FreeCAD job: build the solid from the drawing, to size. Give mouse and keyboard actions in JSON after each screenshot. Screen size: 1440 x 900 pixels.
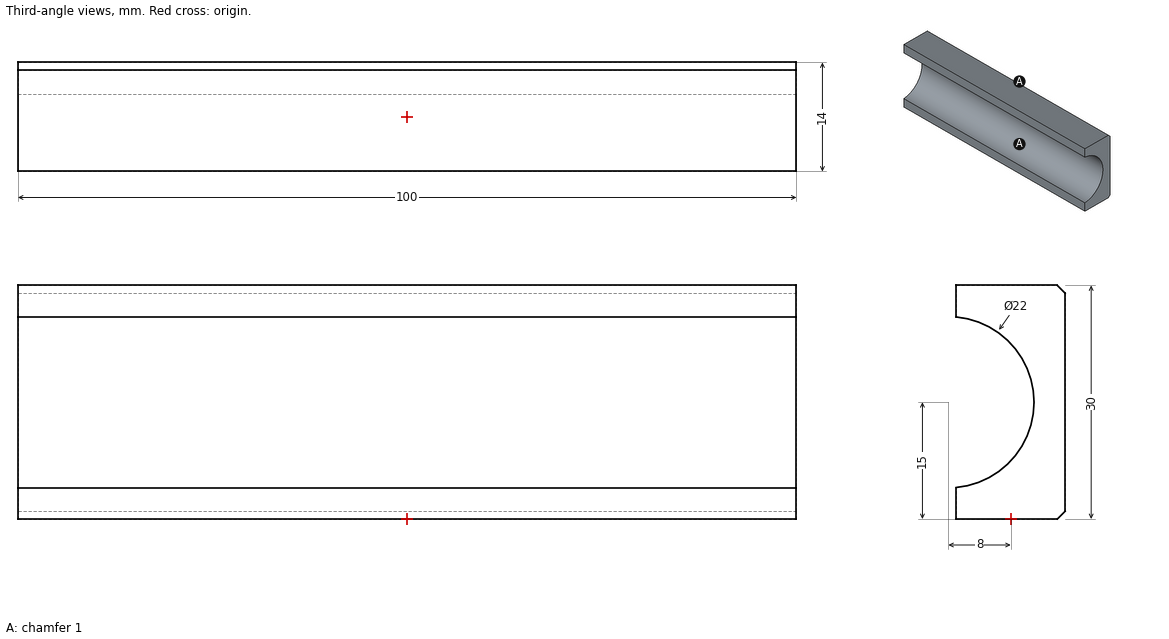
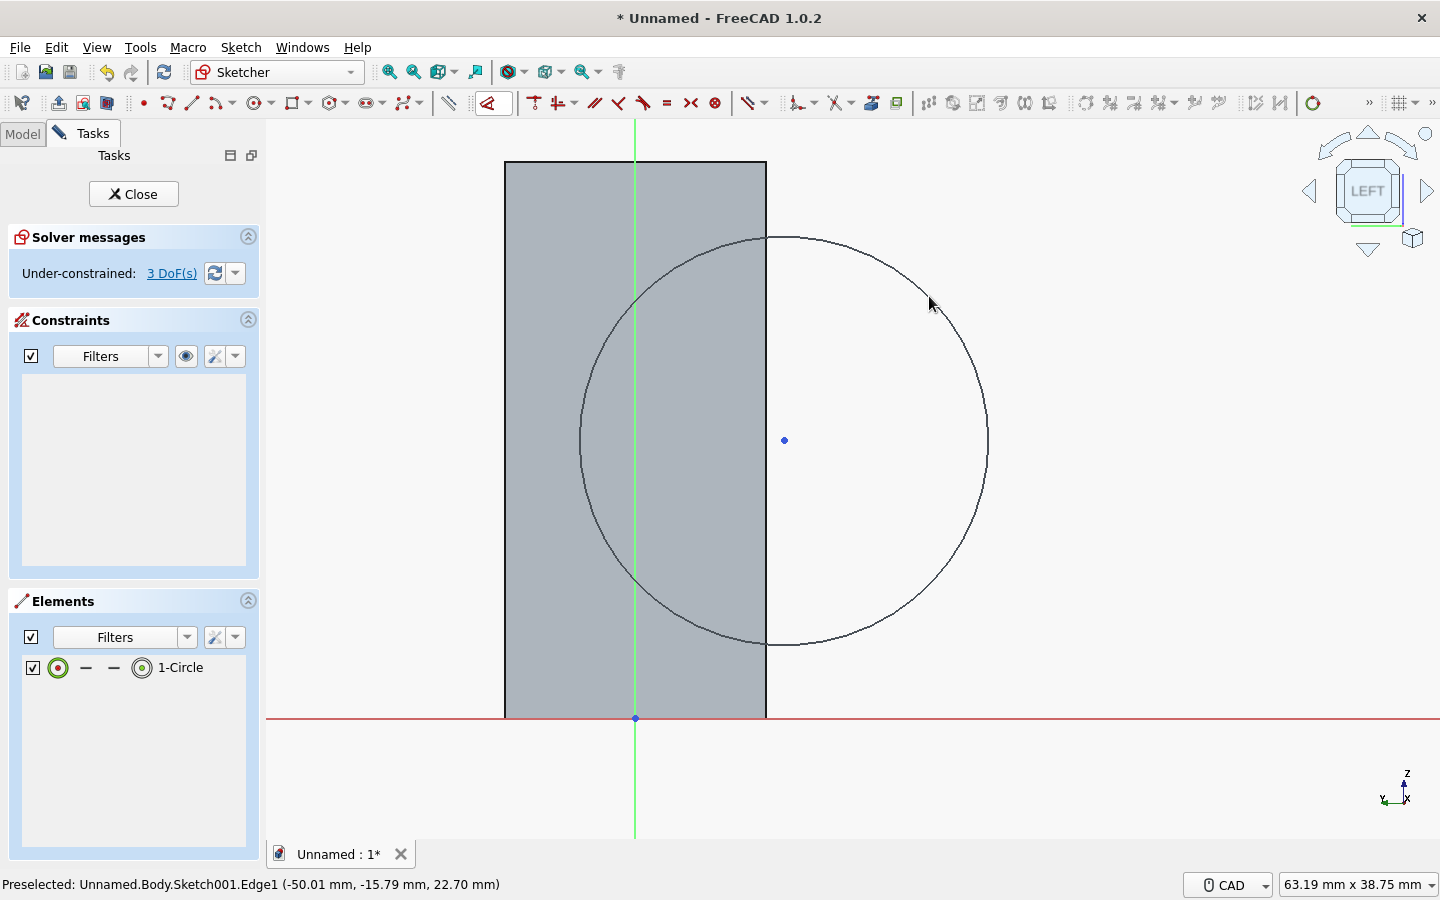
{"action": "left_click", "coordinate": [928, 296]}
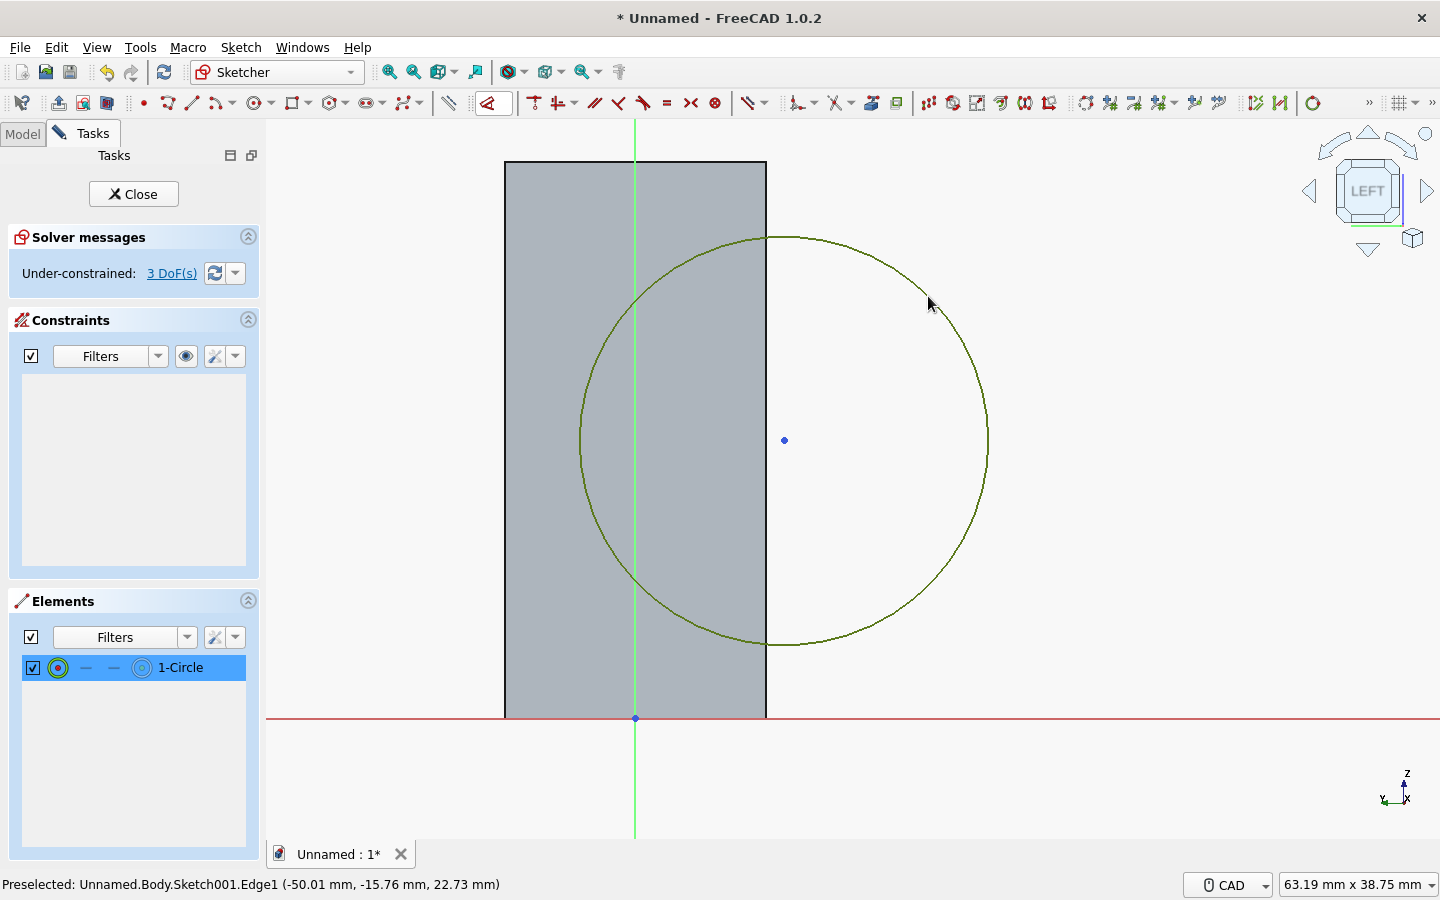
{"action": "key", "text": "k o"}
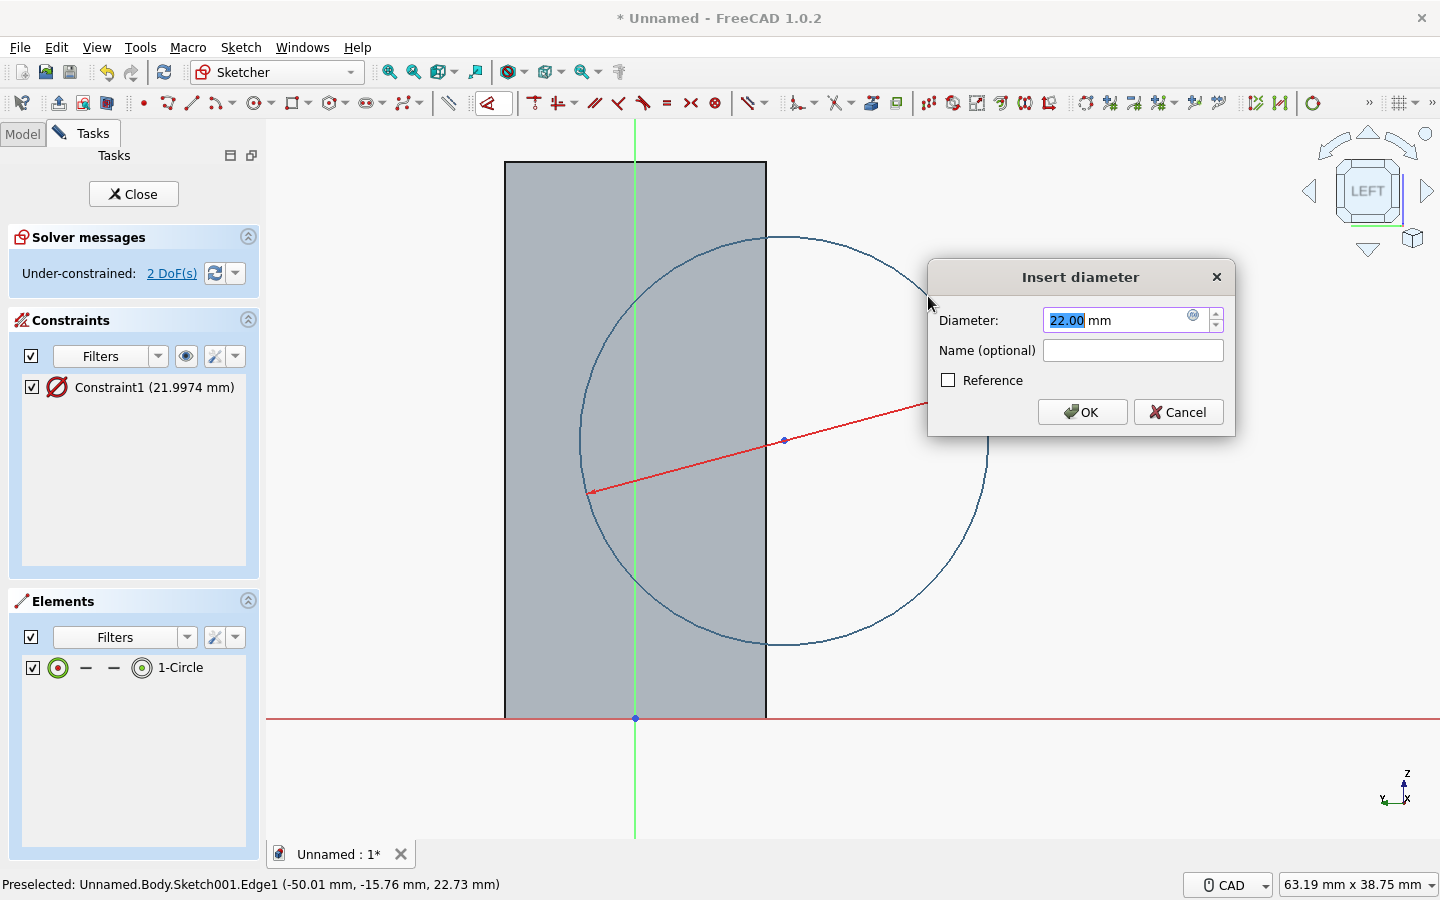
{"action": "type", "text": "22"}
{"action": "key", "text": "Return"}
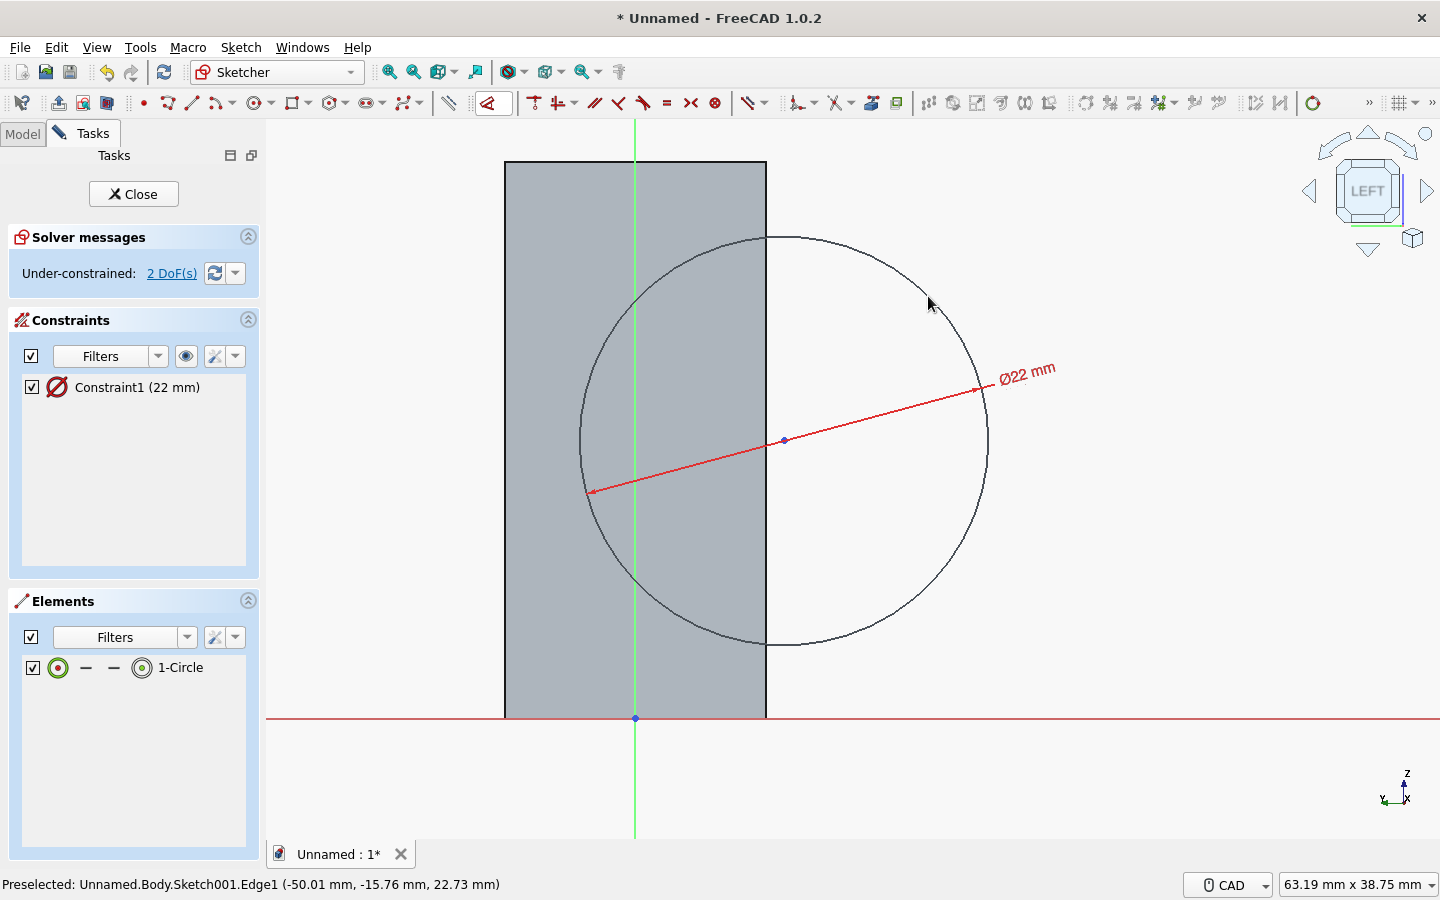
{"action": "left_click", "coordinate": [784, 441]}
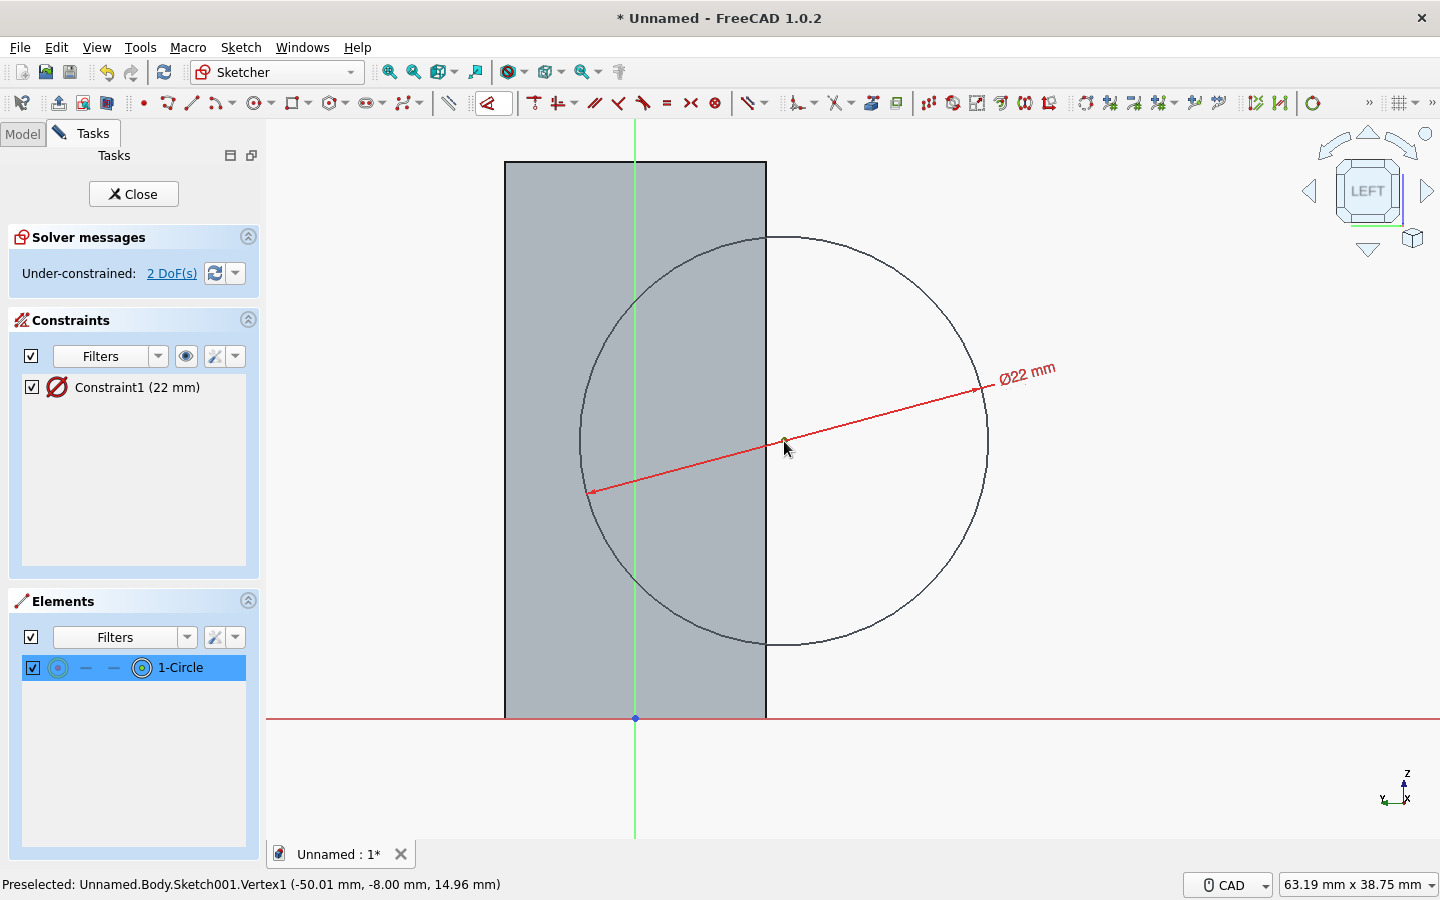
{"action": "left_click", "coordinate": [506, 104]}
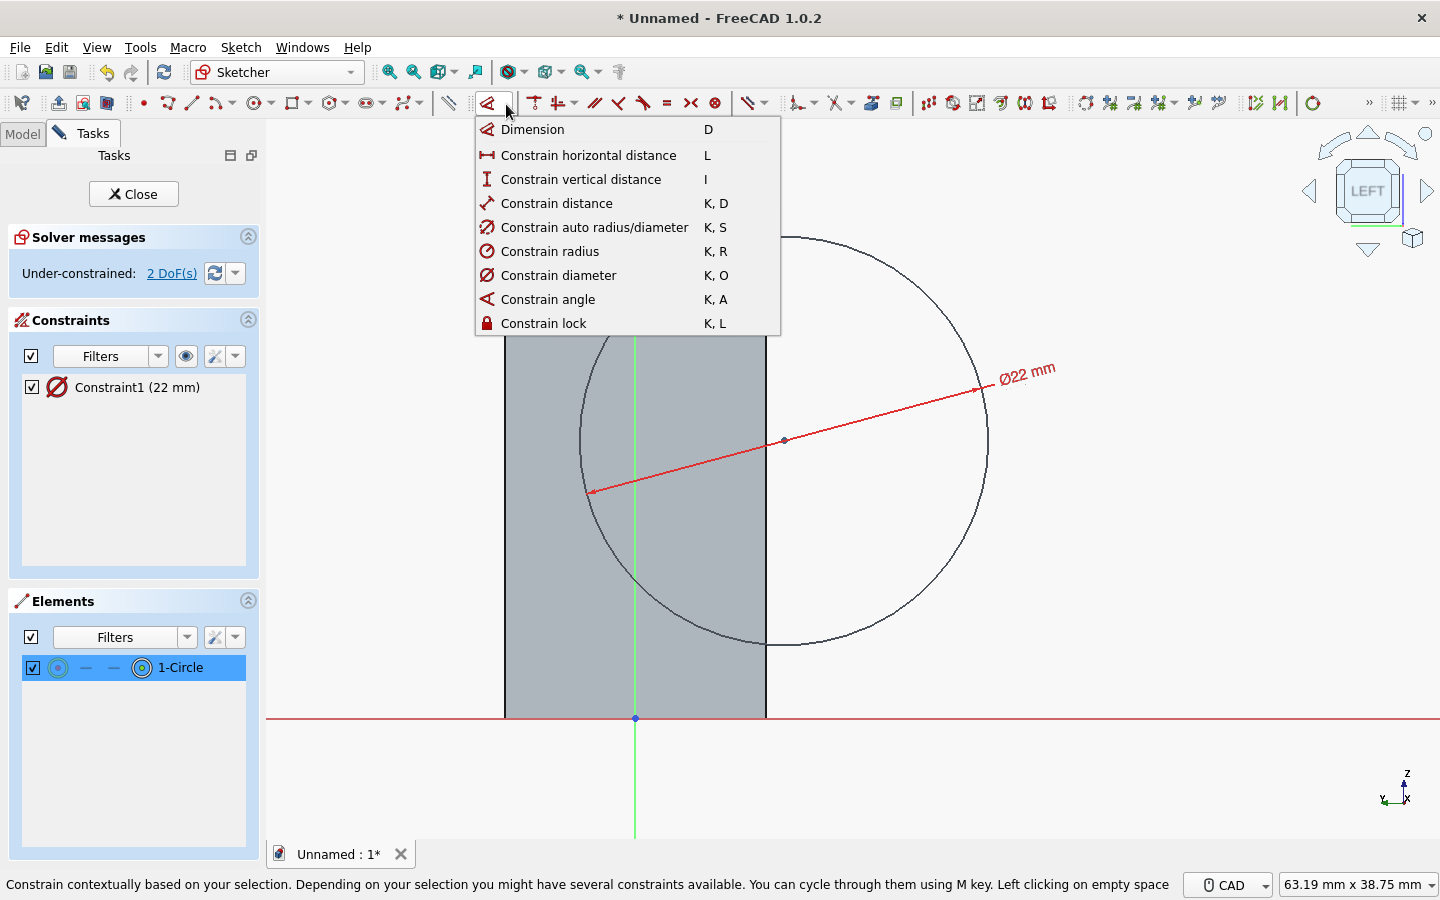
{"action": "left_click", "coordinate": [628, 155]}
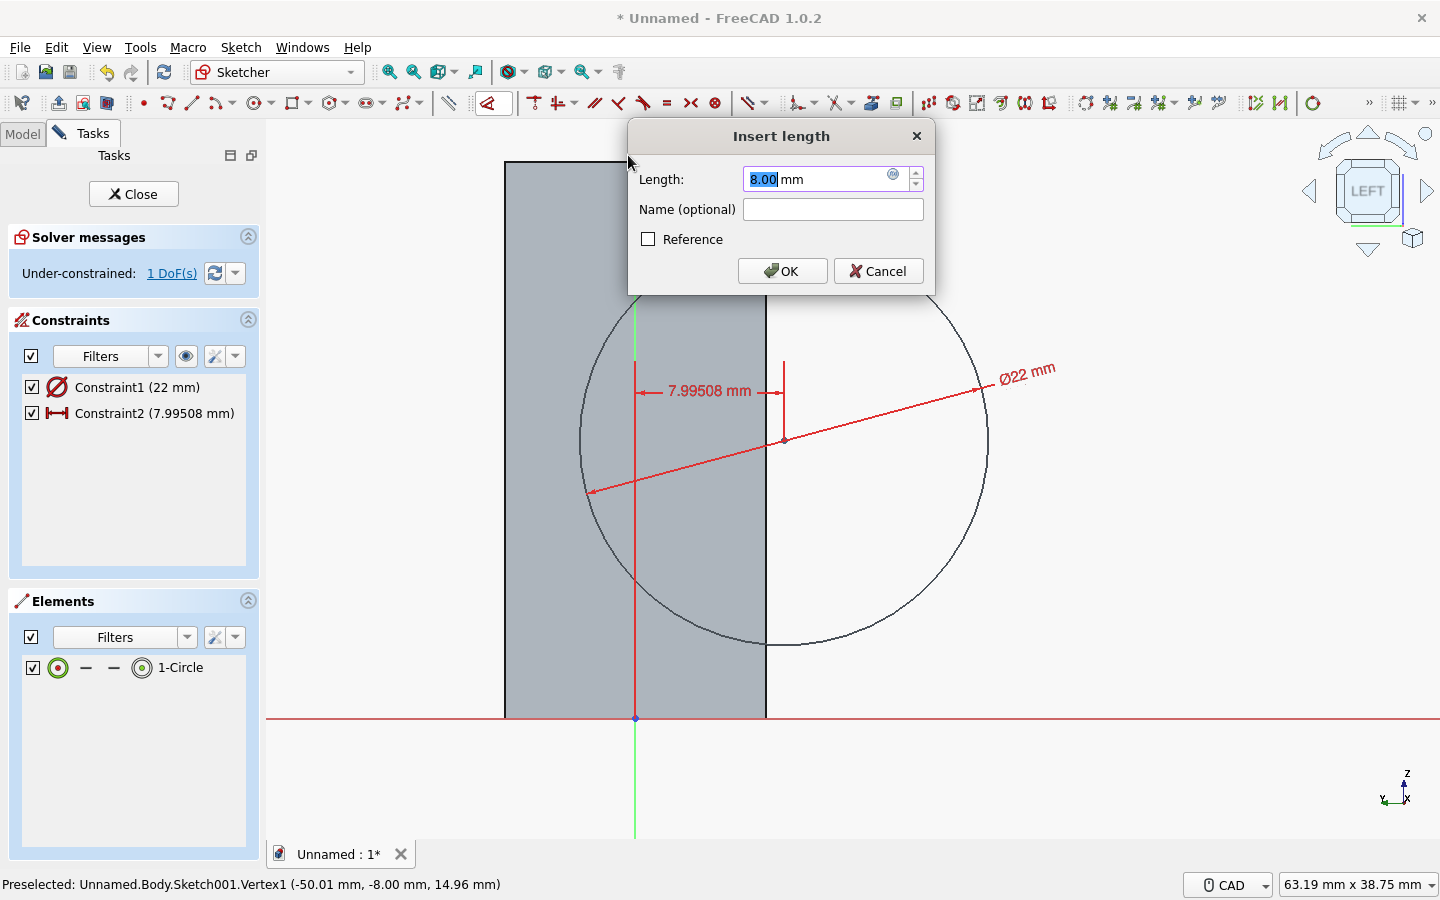
{"action": "type", "text": "8"}
{"action": "key", "text": "Return"}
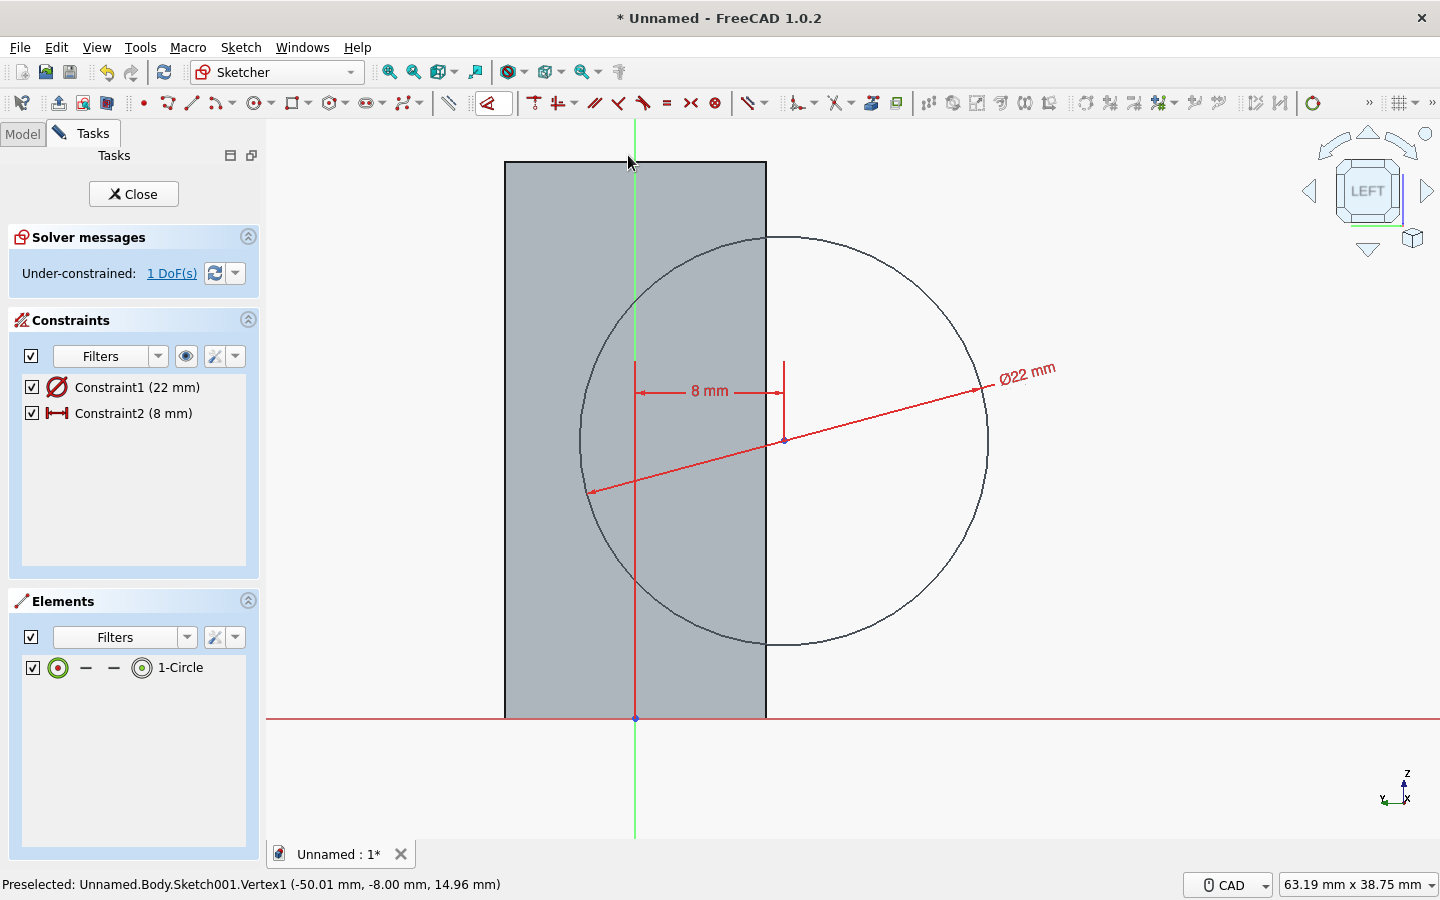
{"action": "left_click", "coordinate": [784, 441]}